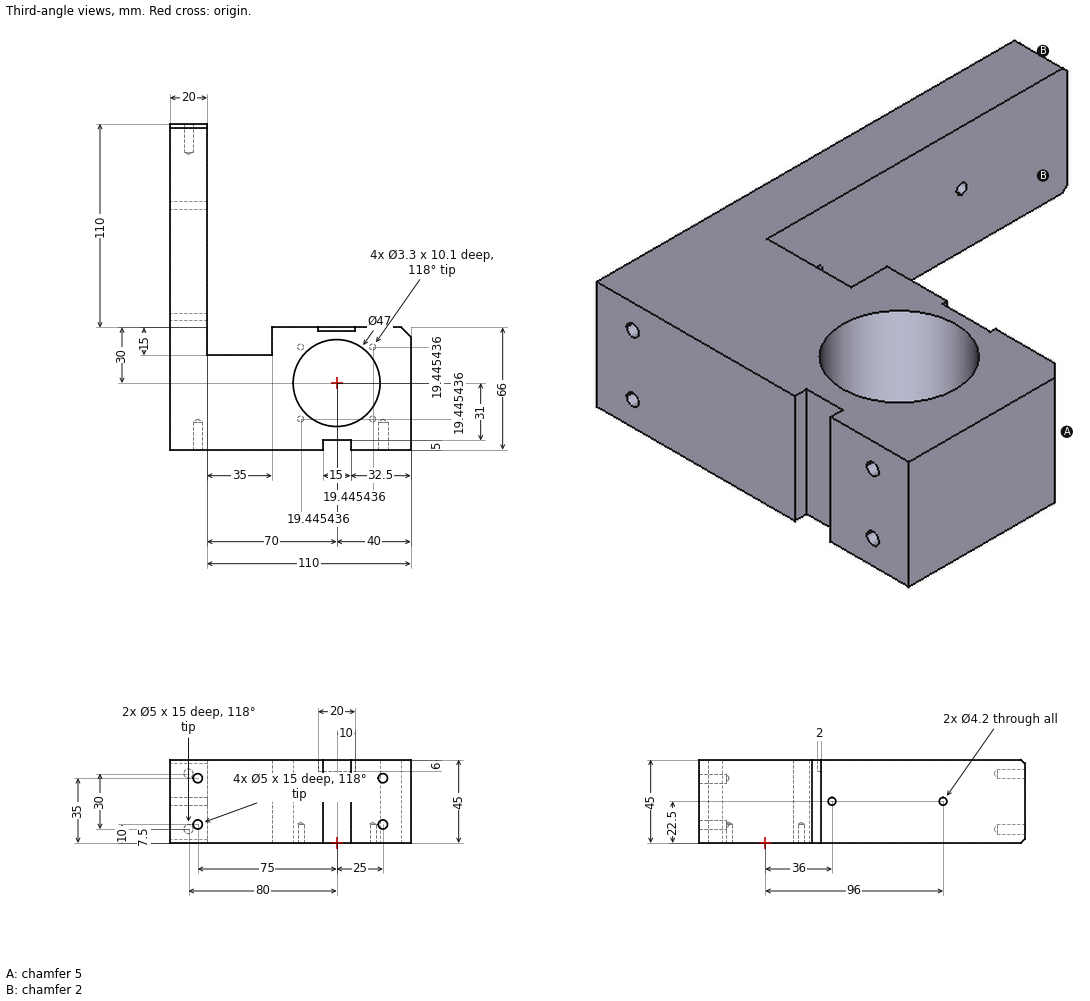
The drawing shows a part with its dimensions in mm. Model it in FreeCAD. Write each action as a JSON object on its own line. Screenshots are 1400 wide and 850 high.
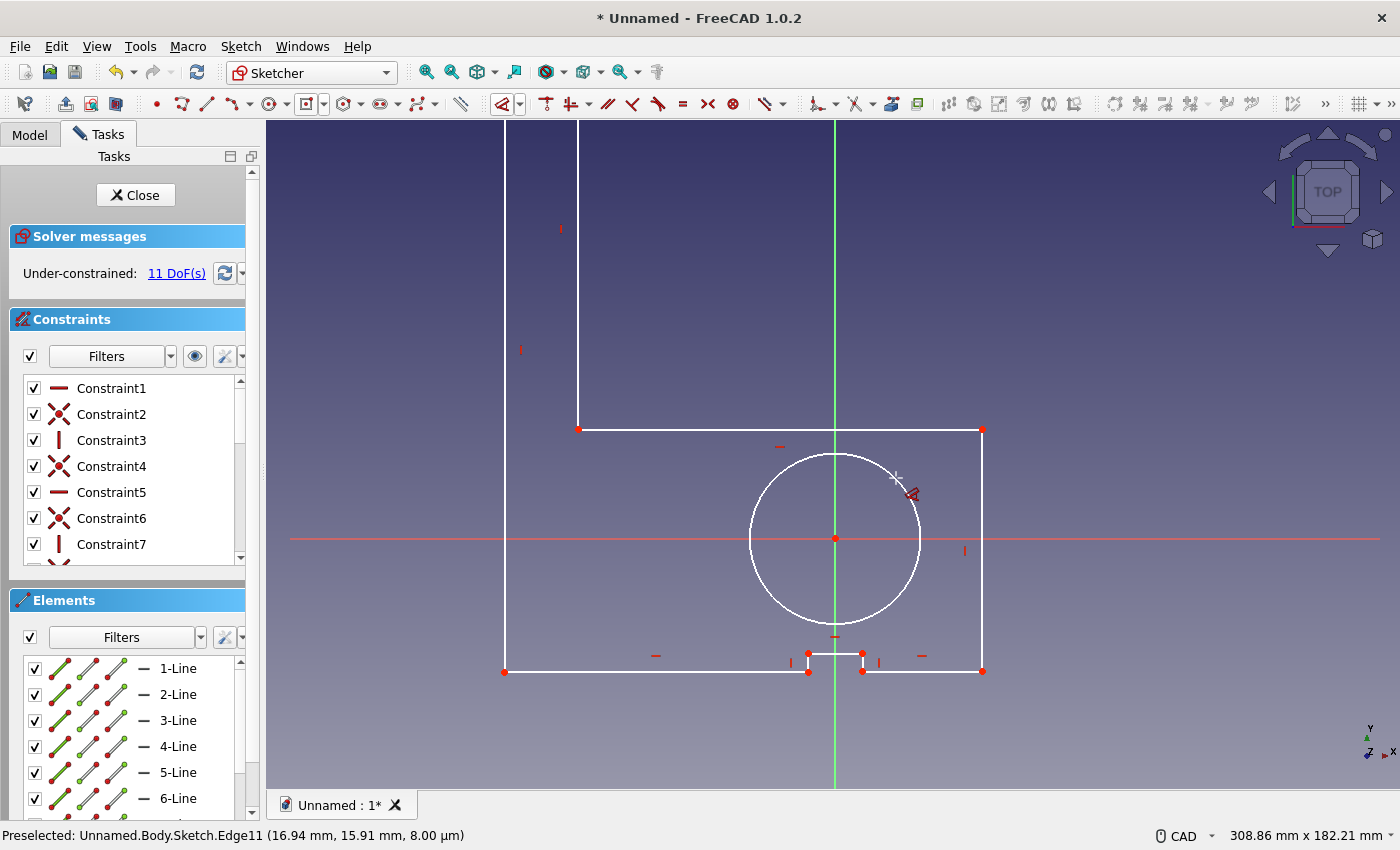
{"action": "left_click", "coordinate": [895, 478]}
{"action": "left_click", "coordinate": [917, 455]}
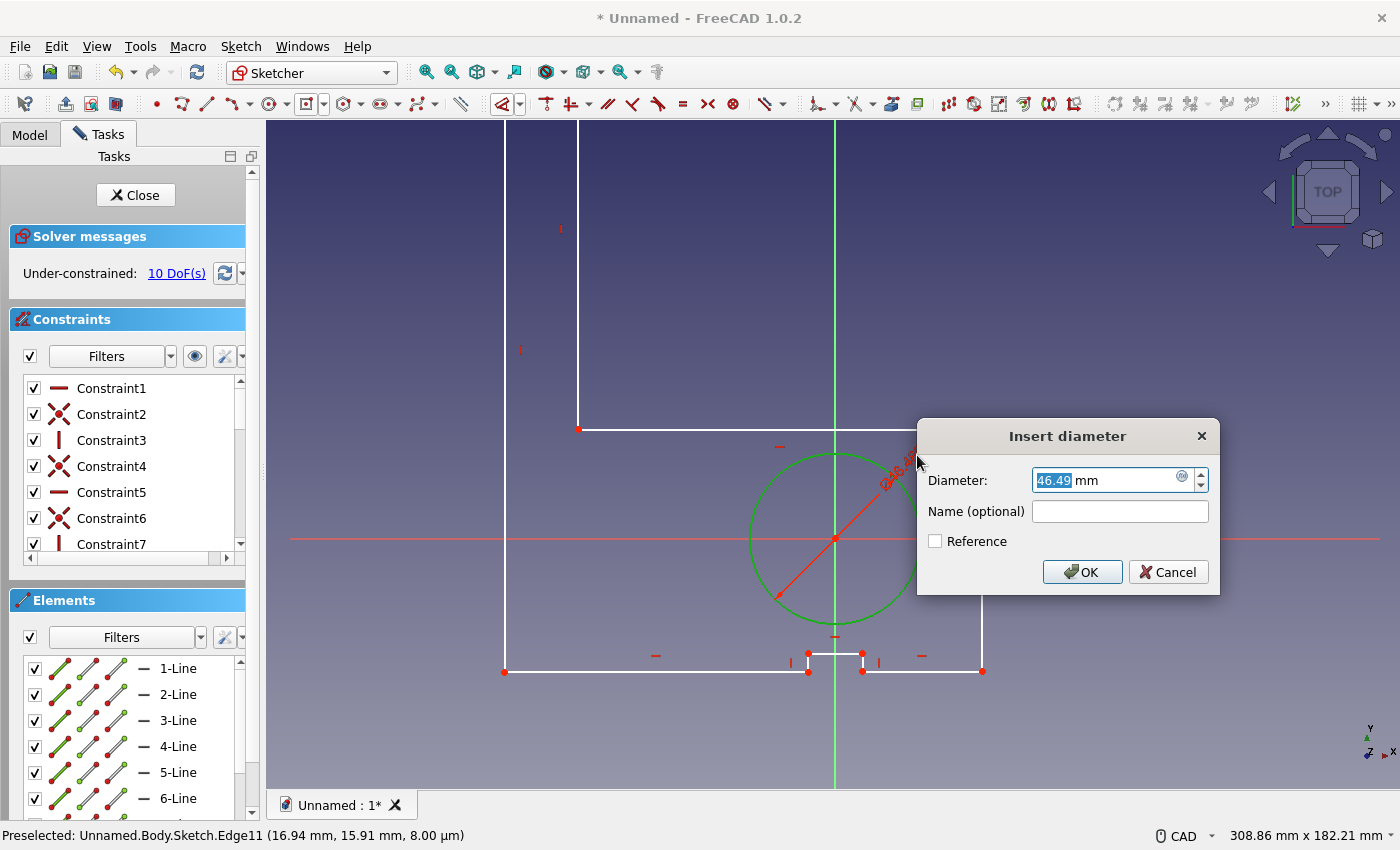
{"action": "type", "text": "47"}
{"action": "key", "text": "Return"}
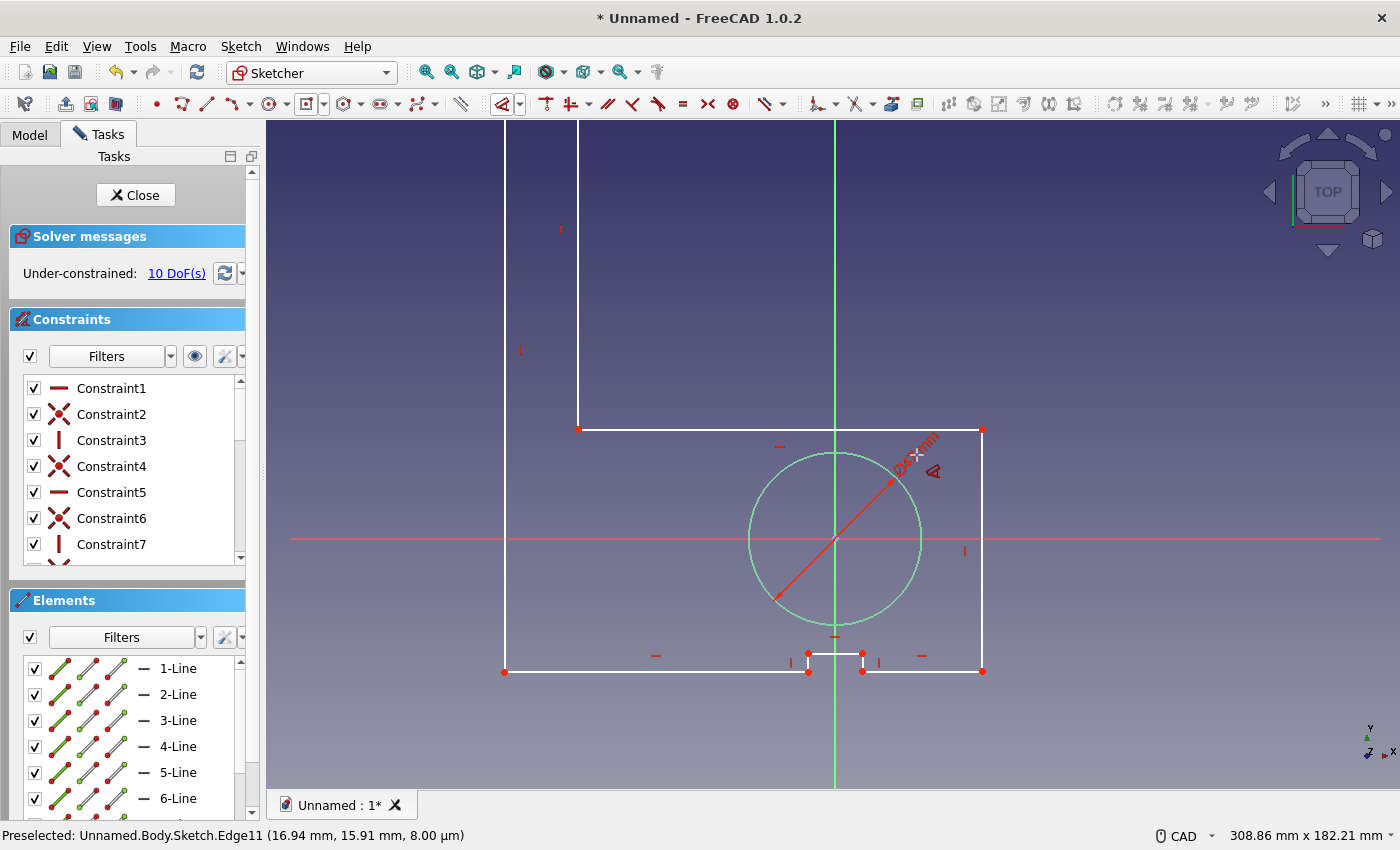
{"action": "scroll", "coordinate": [863, 663], "scroll_direction": "up", "scroll_amount": 4}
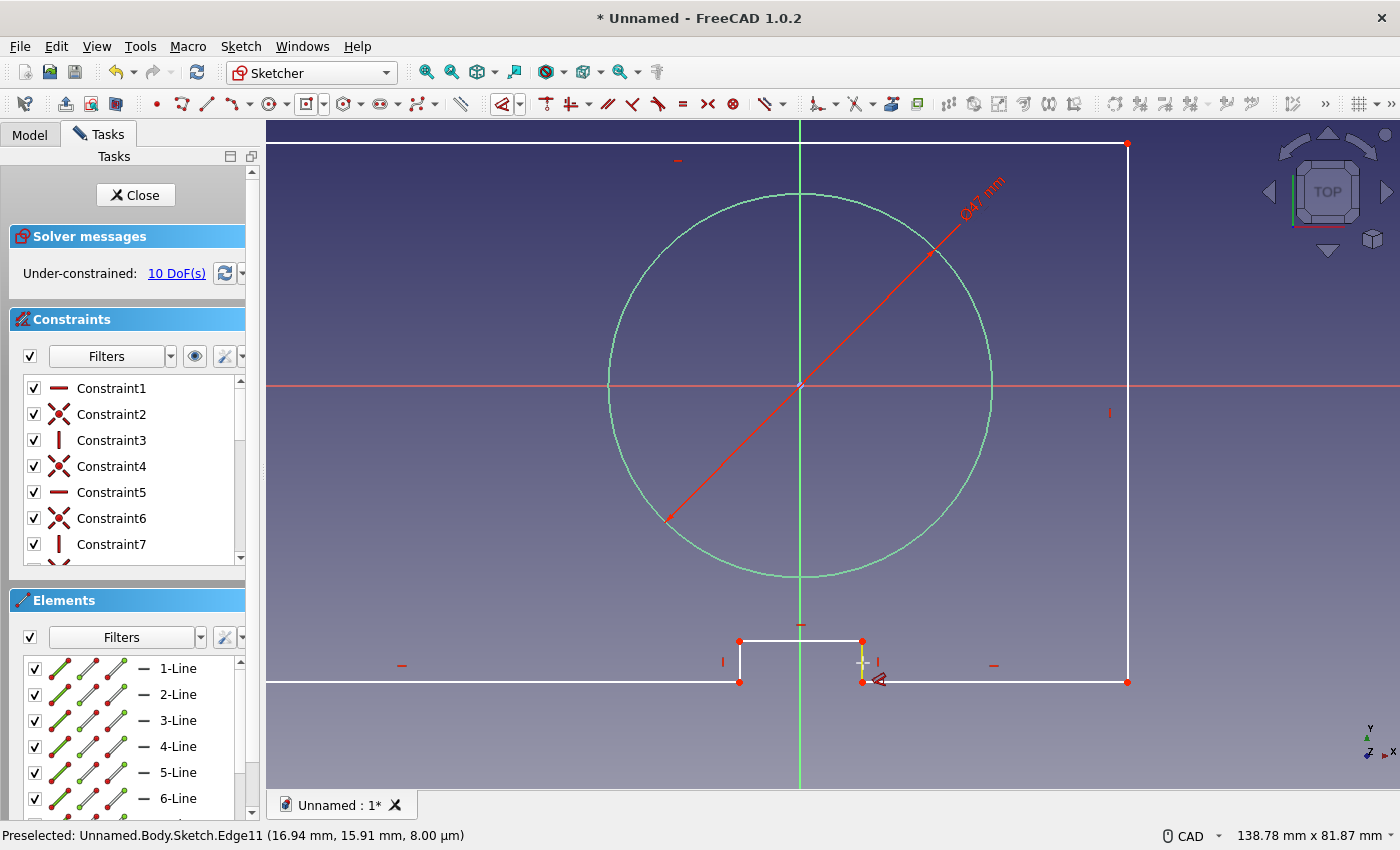
{"action": "left_click", "coordinate": [862, 662]}
{"action": "left_click", "coordinate": [896, 662]}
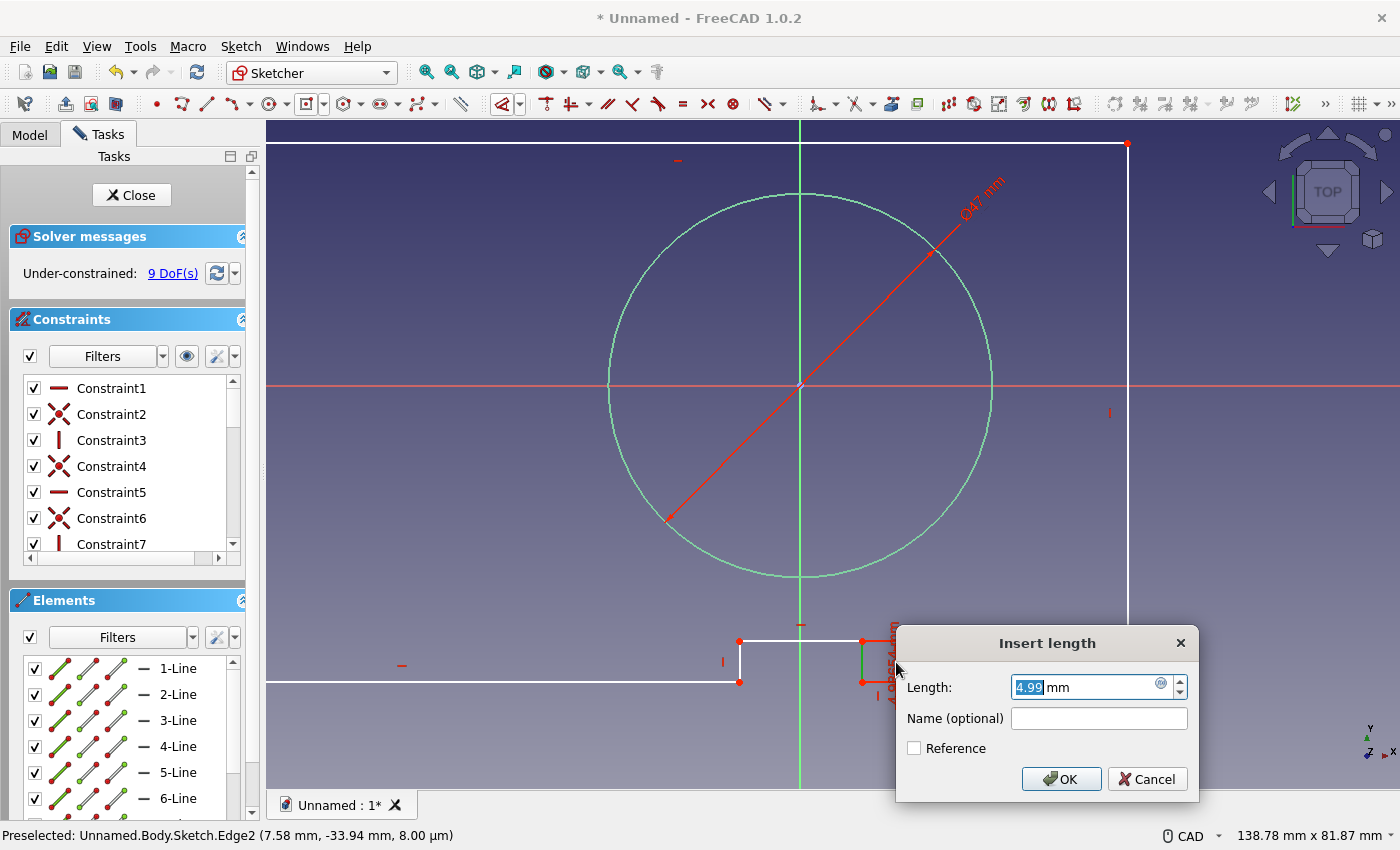
{"action": "type", "text": "5"}
{"action": "key", "text": "Return"}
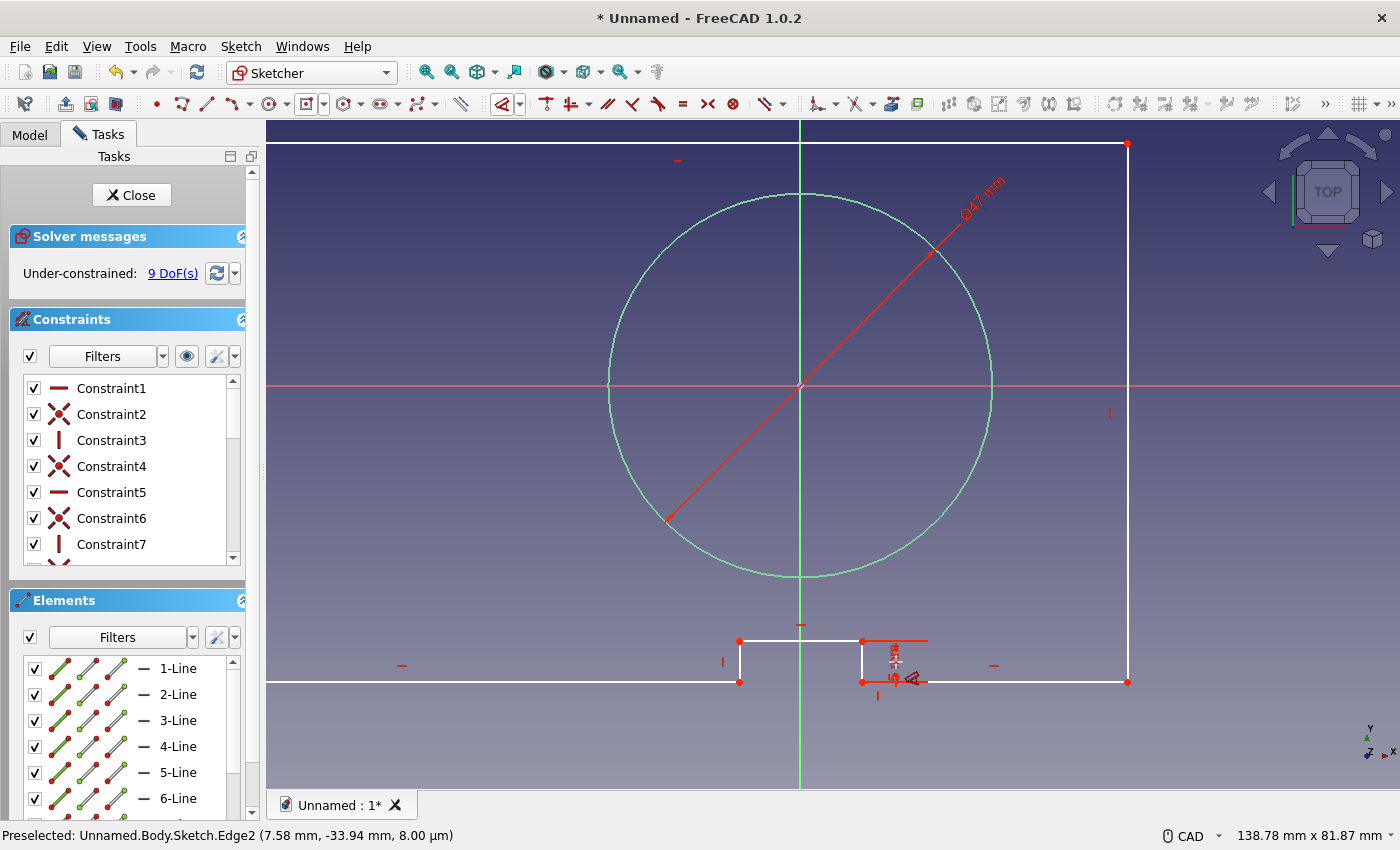
{"action": "left_click", "coordinate": [740, 670]}
{"action": "left_click", "coordinate": [774, 662]}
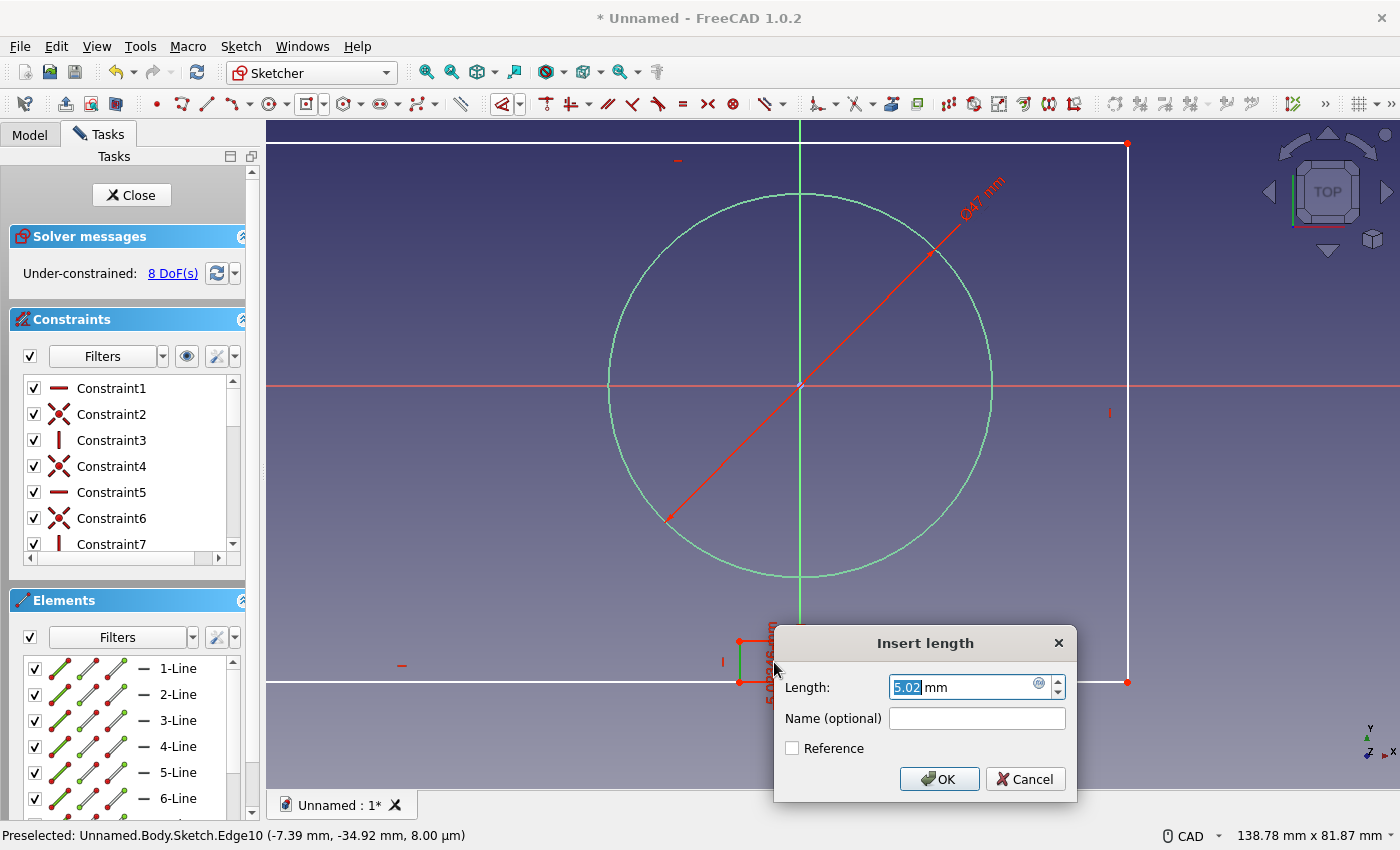
{"action": "type", "text": "5"}
{"action": "key", "text": "Return"}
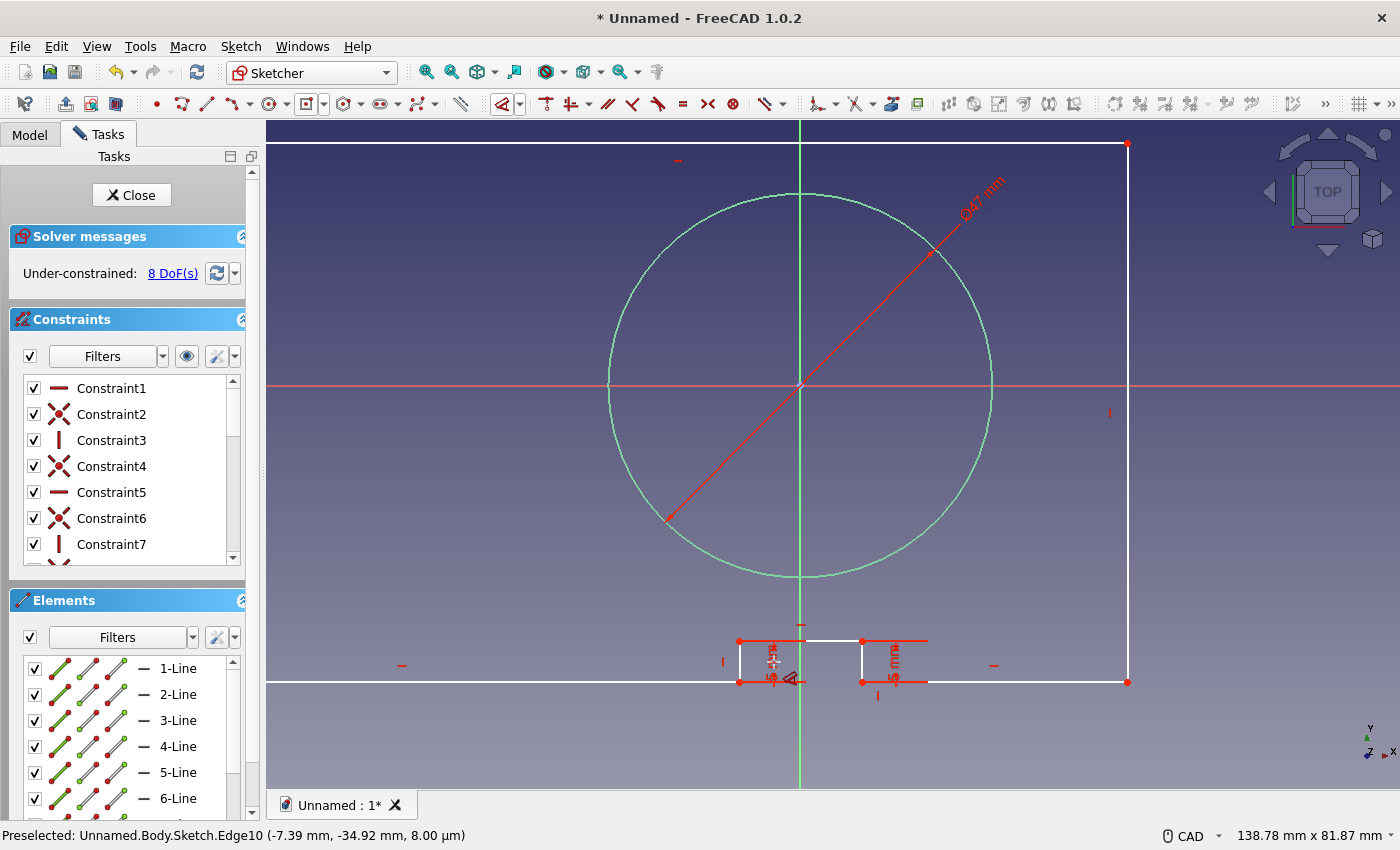
{"action": "left_click", "coordinate": [777, 641]}
{"action": "left_click", "coordinate": [773, 607]}